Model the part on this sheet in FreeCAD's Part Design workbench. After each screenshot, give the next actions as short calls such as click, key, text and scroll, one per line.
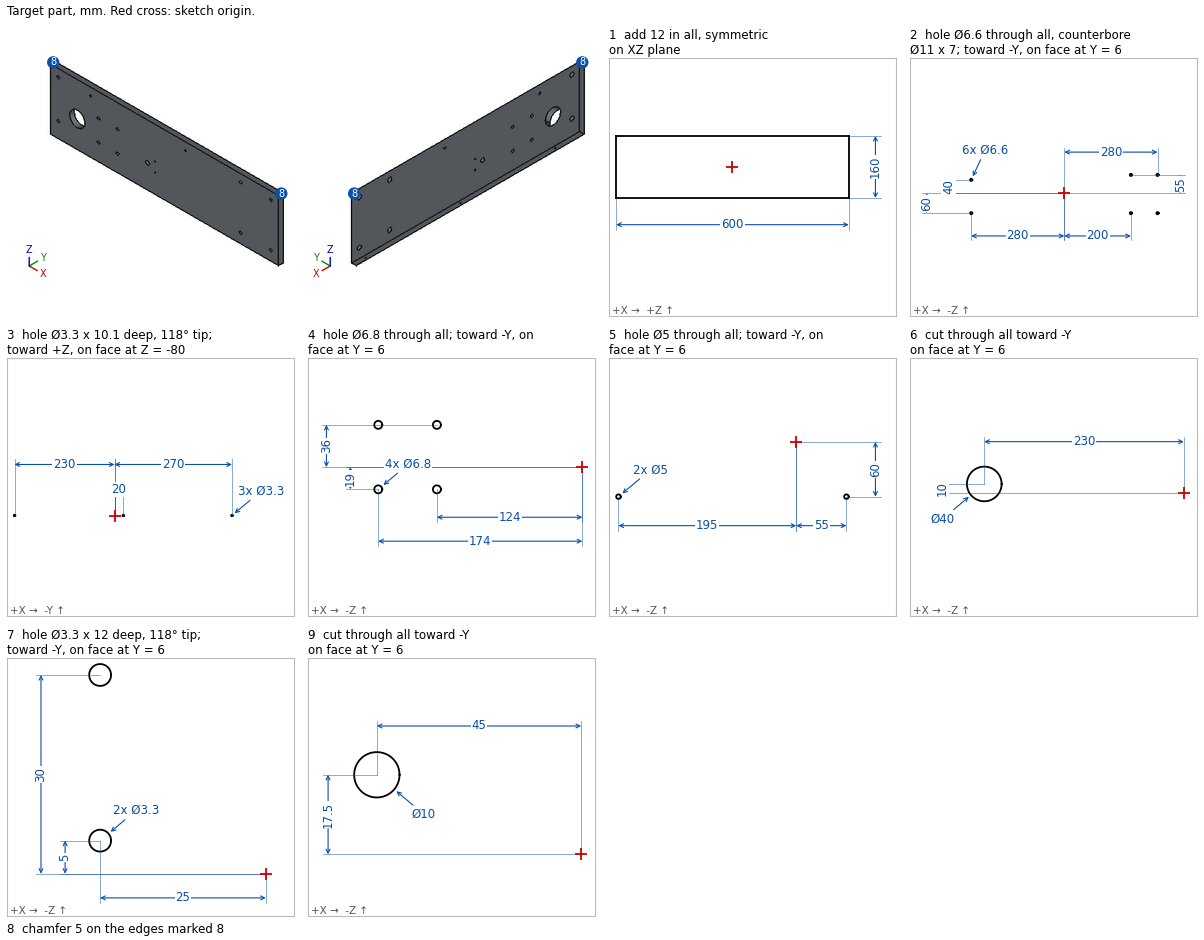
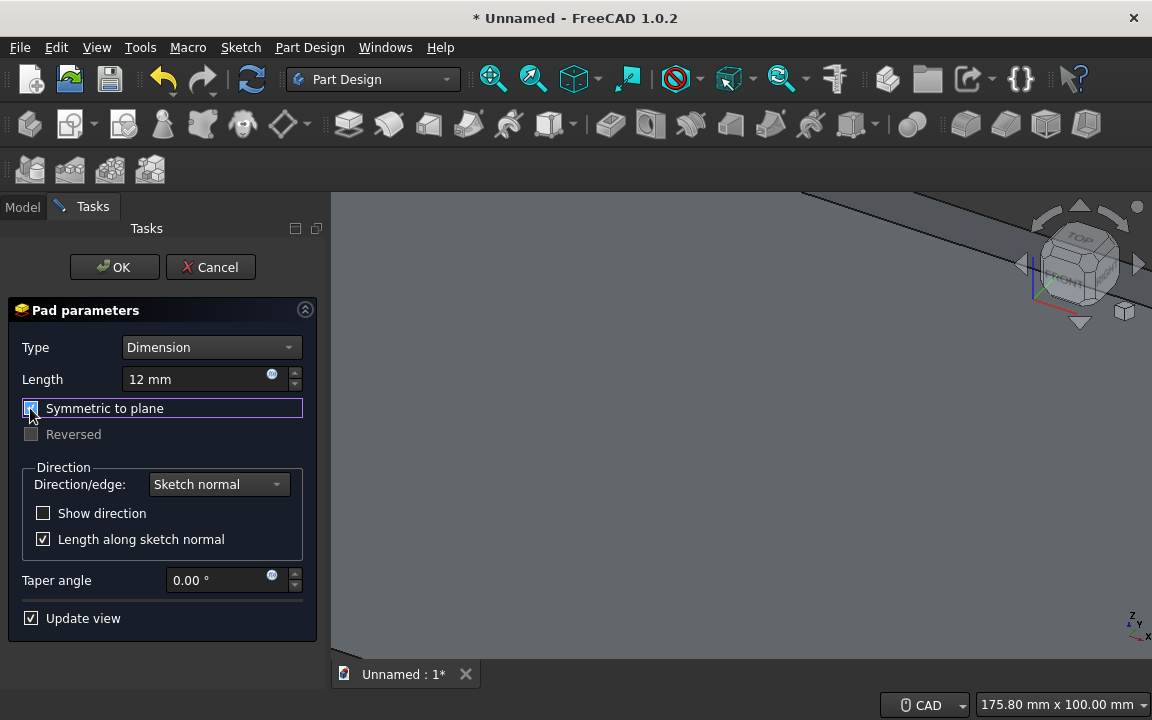
click(115, 267)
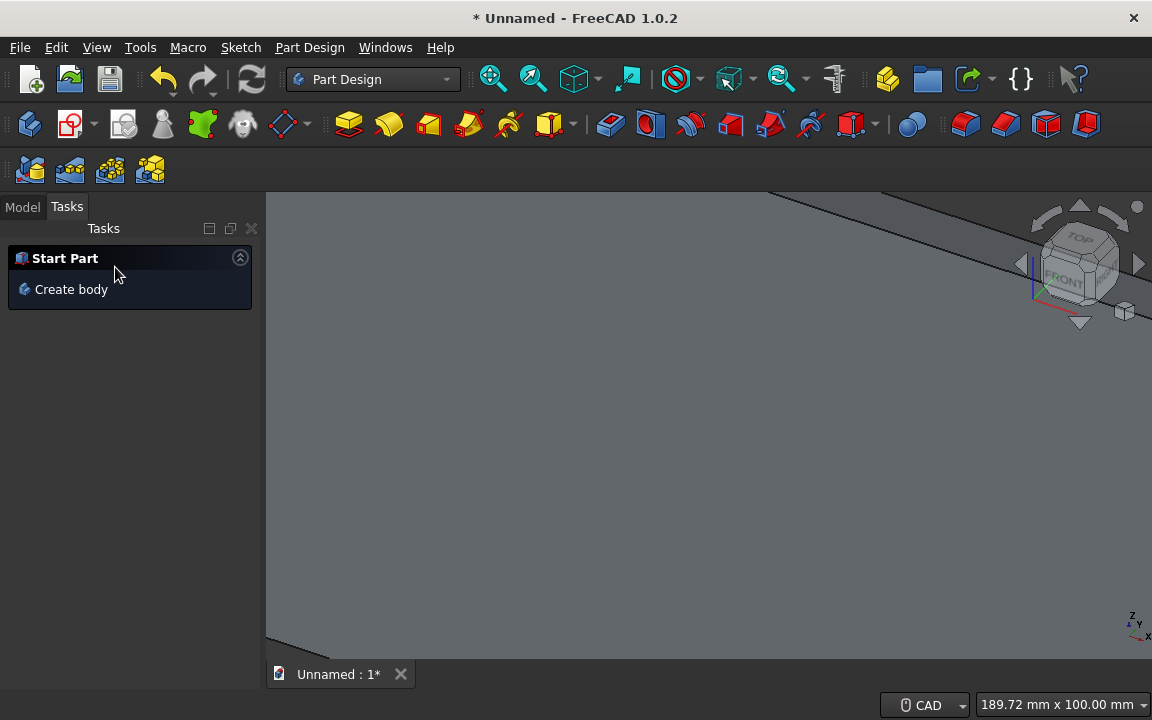
click(494, 80)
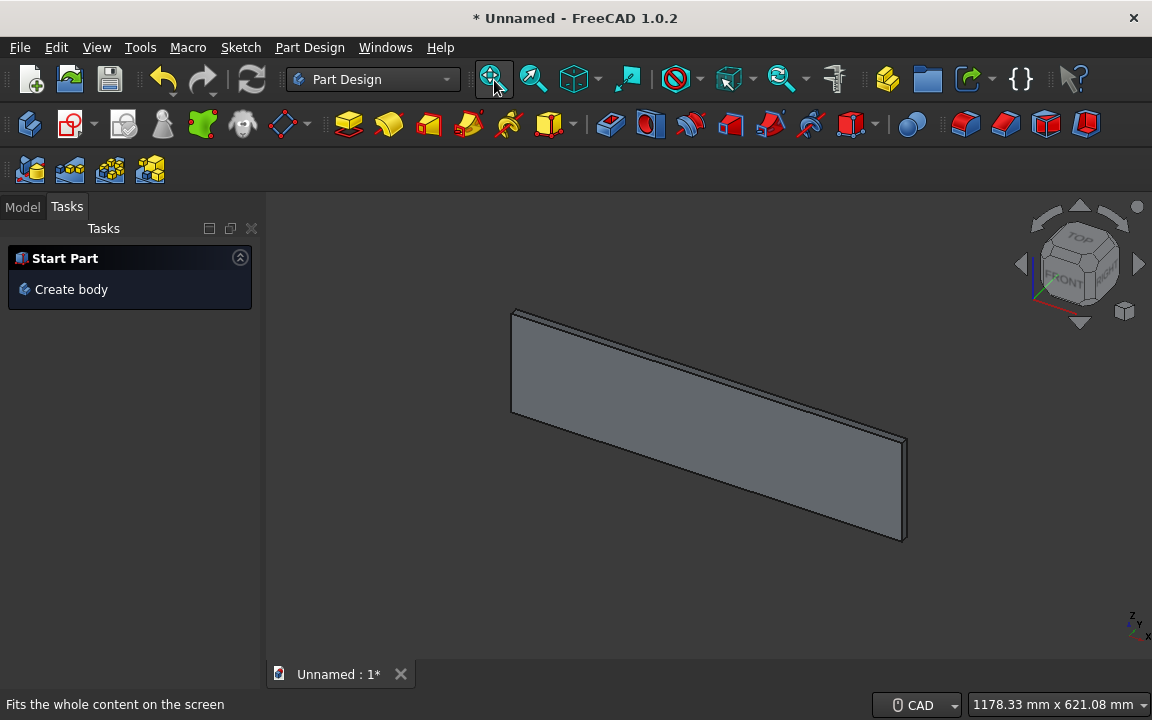
key(4)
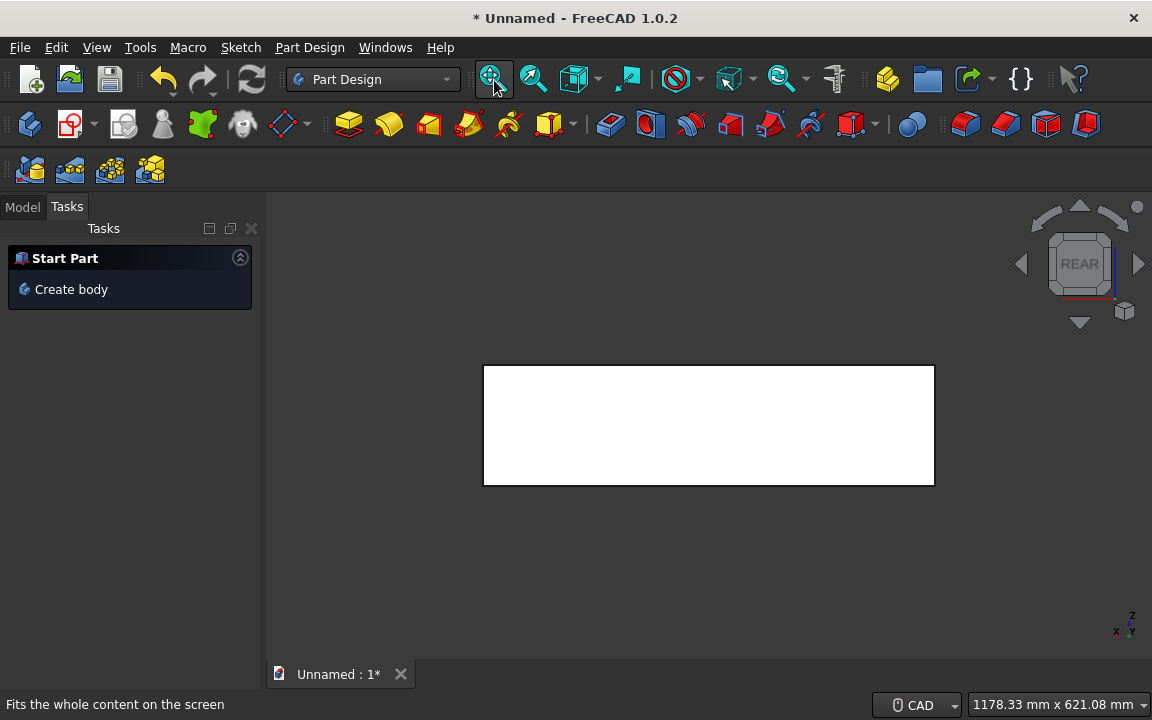
click(580, 424)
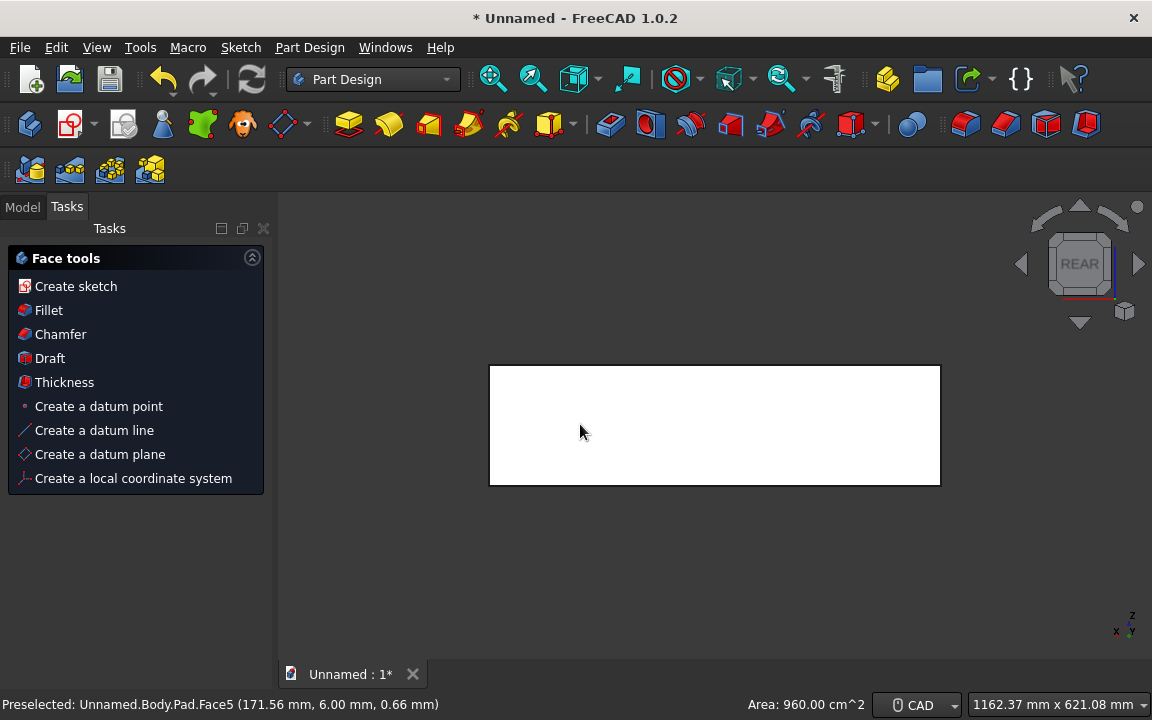
click(70, 124)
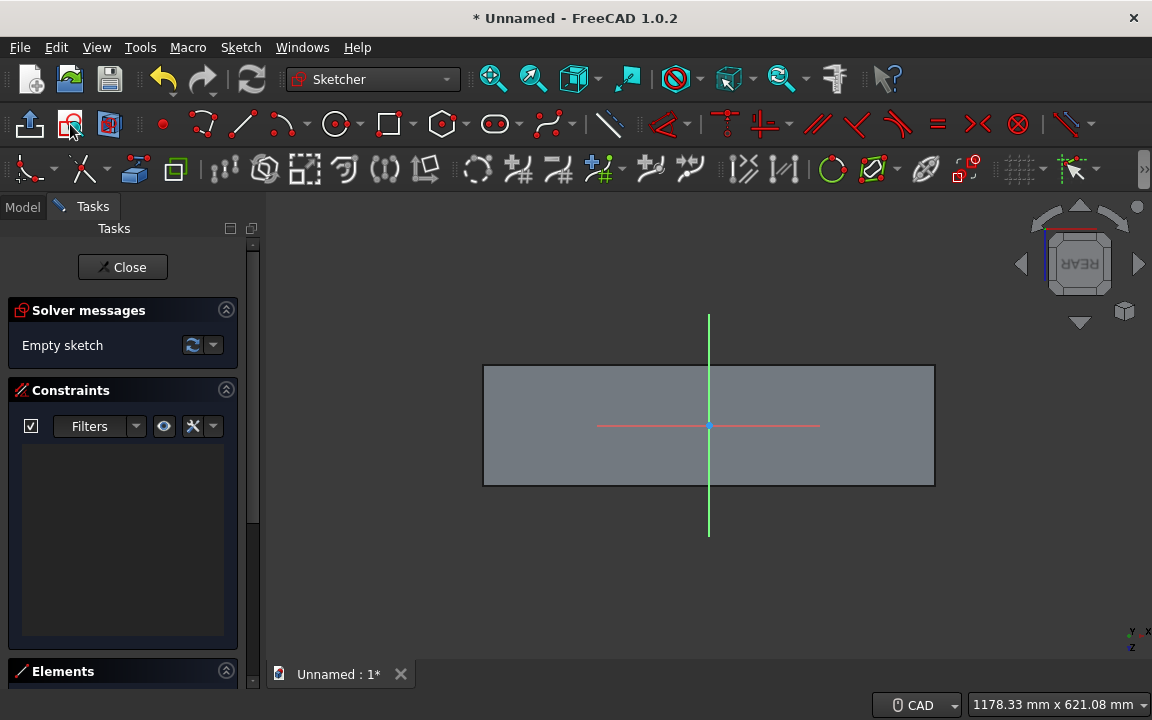
click(336, 124)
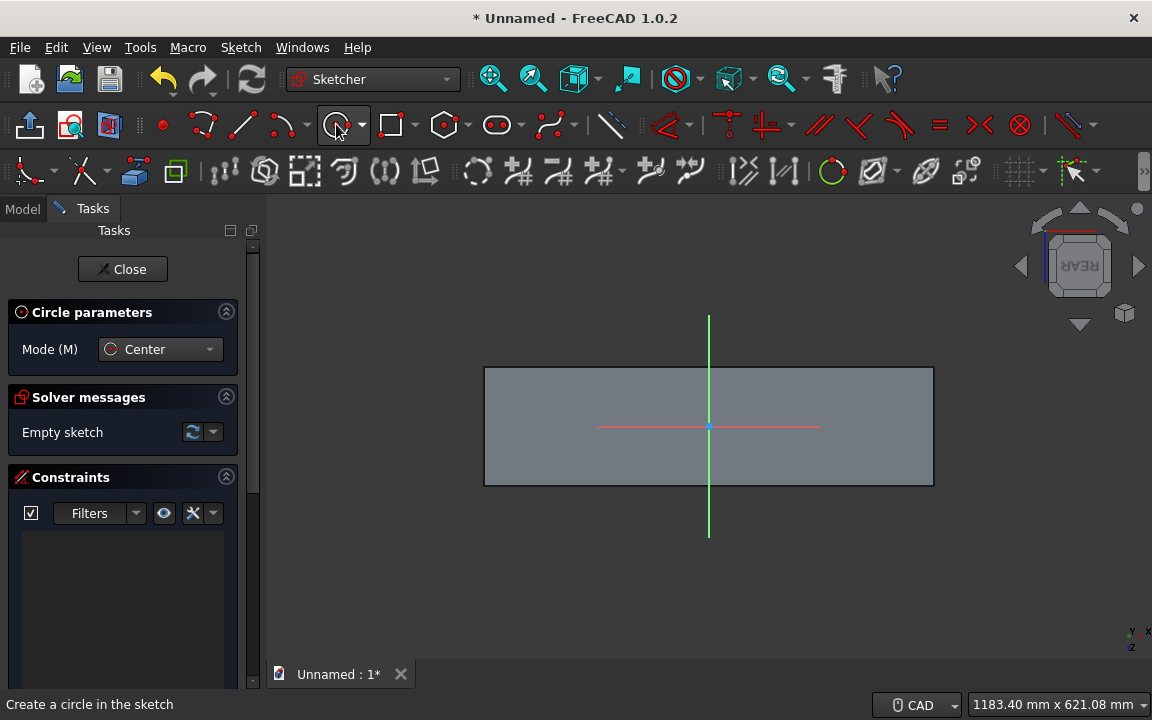
scroll(499, 471, up, 12)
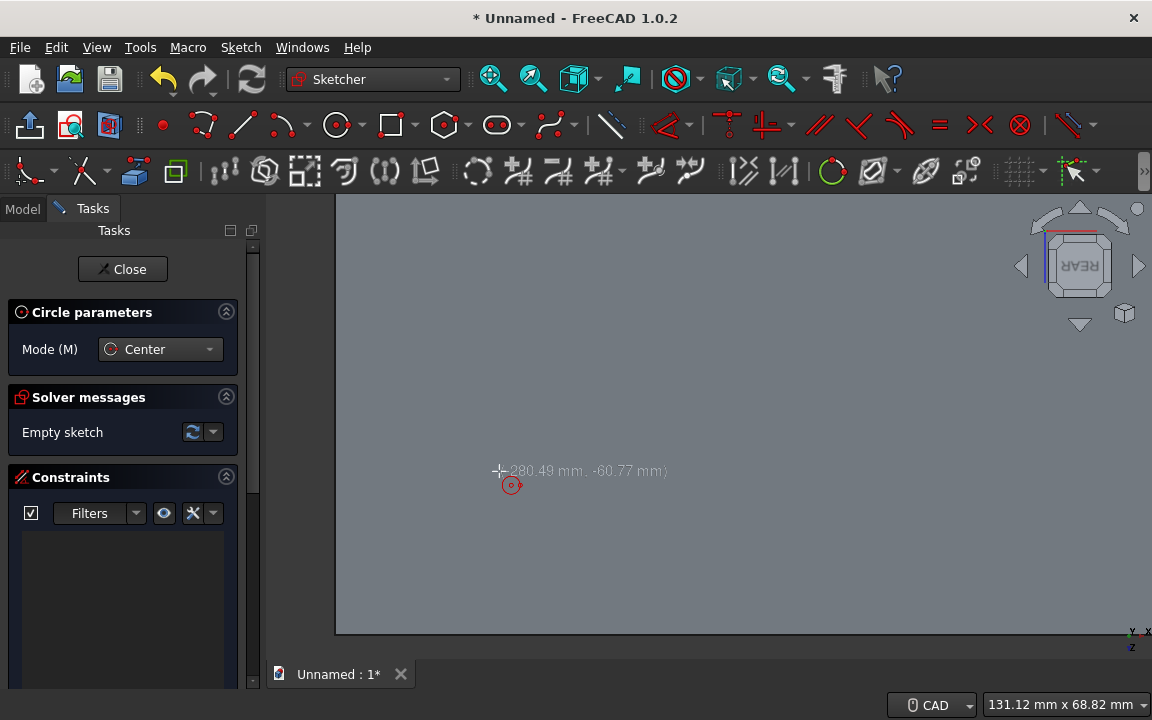
scroll(370, 480, down, 11)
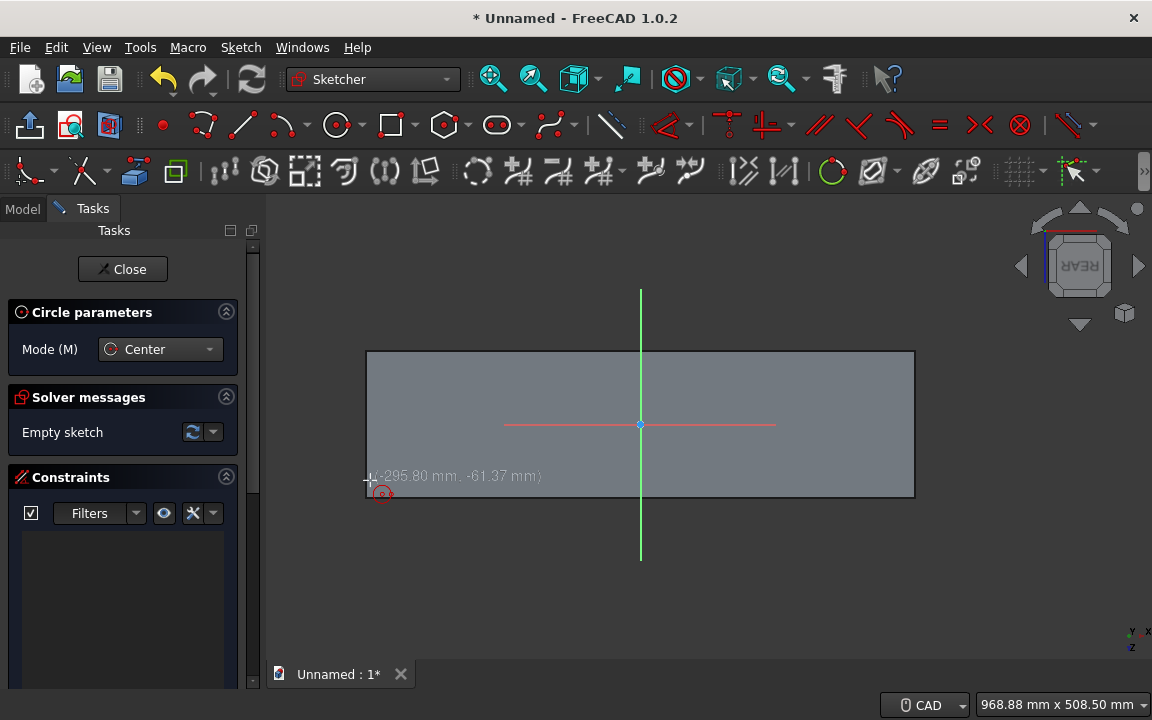
click(385, 479)
move(387, 477)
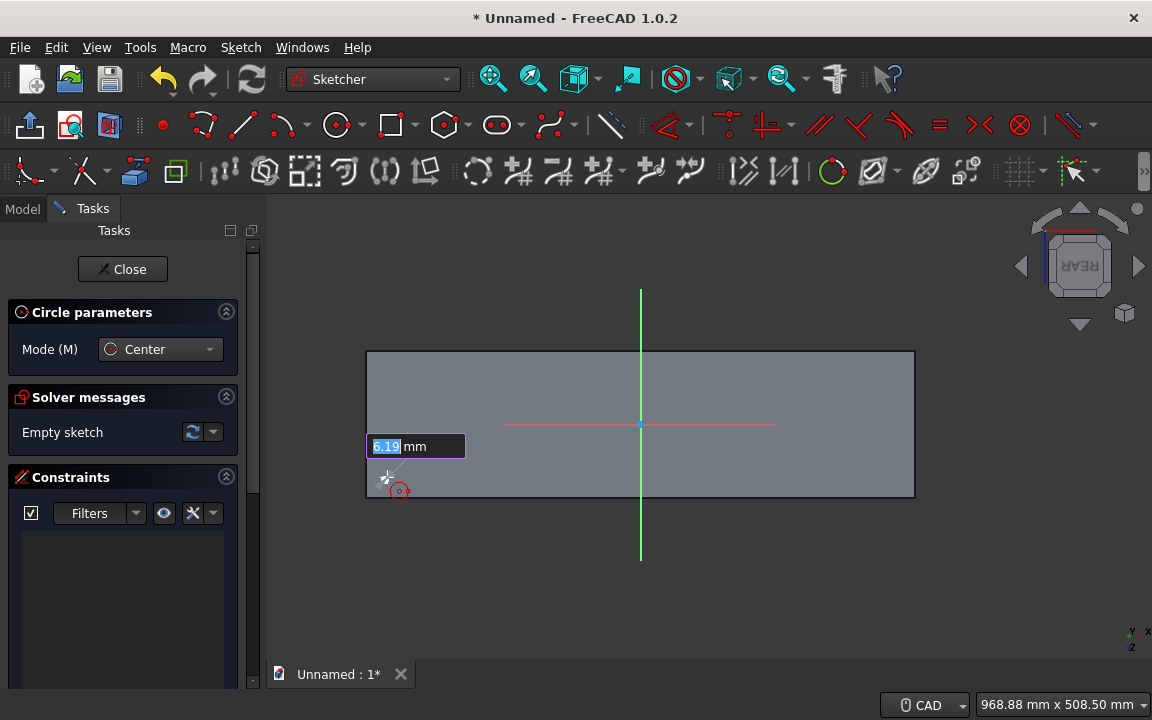
text(6.6)
key(Return)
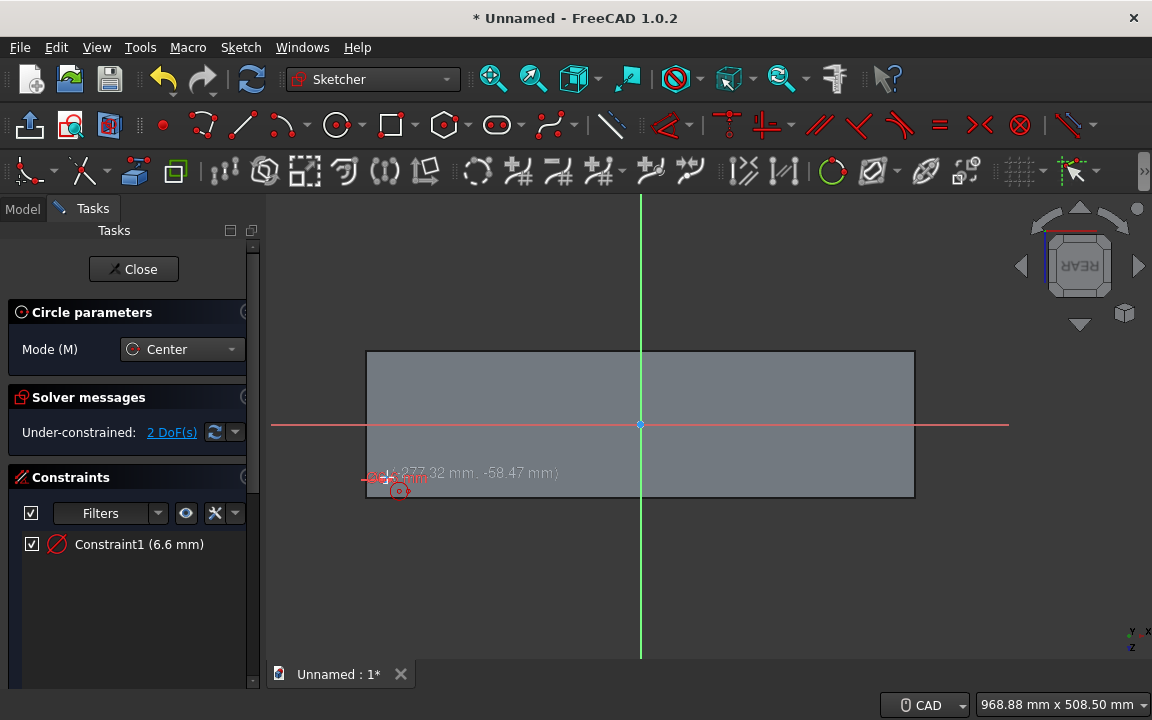
scroll(385, 388, up, 11)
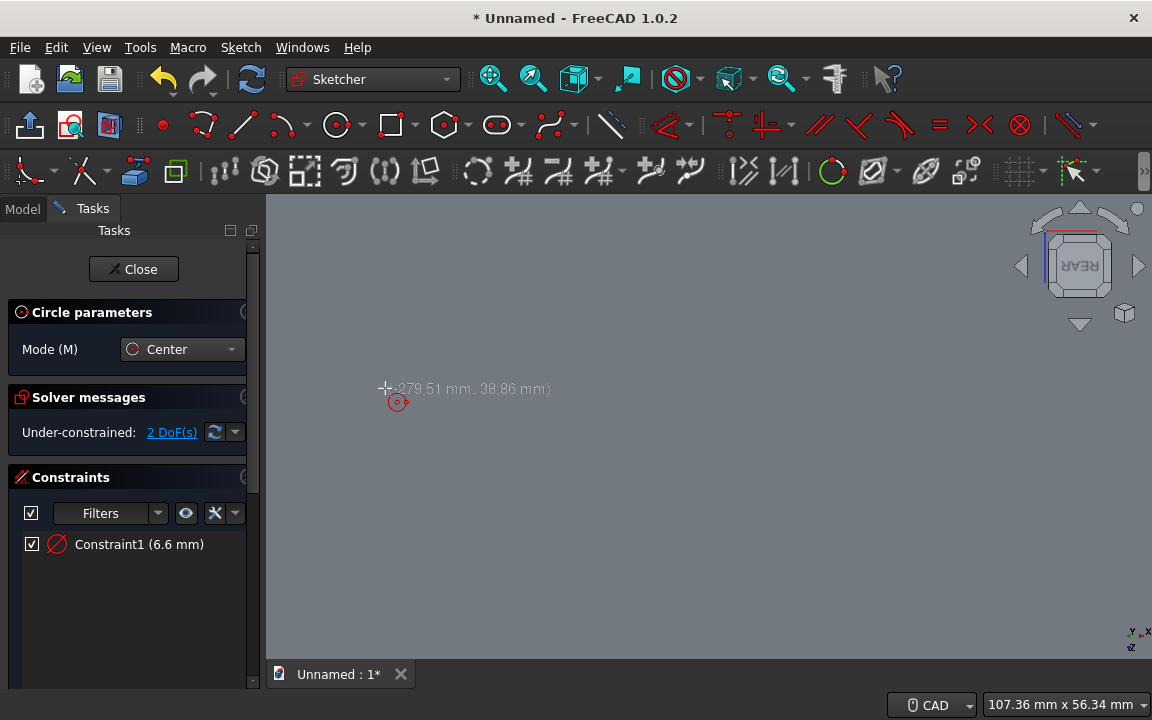
scroll(385, 388, down, 11)